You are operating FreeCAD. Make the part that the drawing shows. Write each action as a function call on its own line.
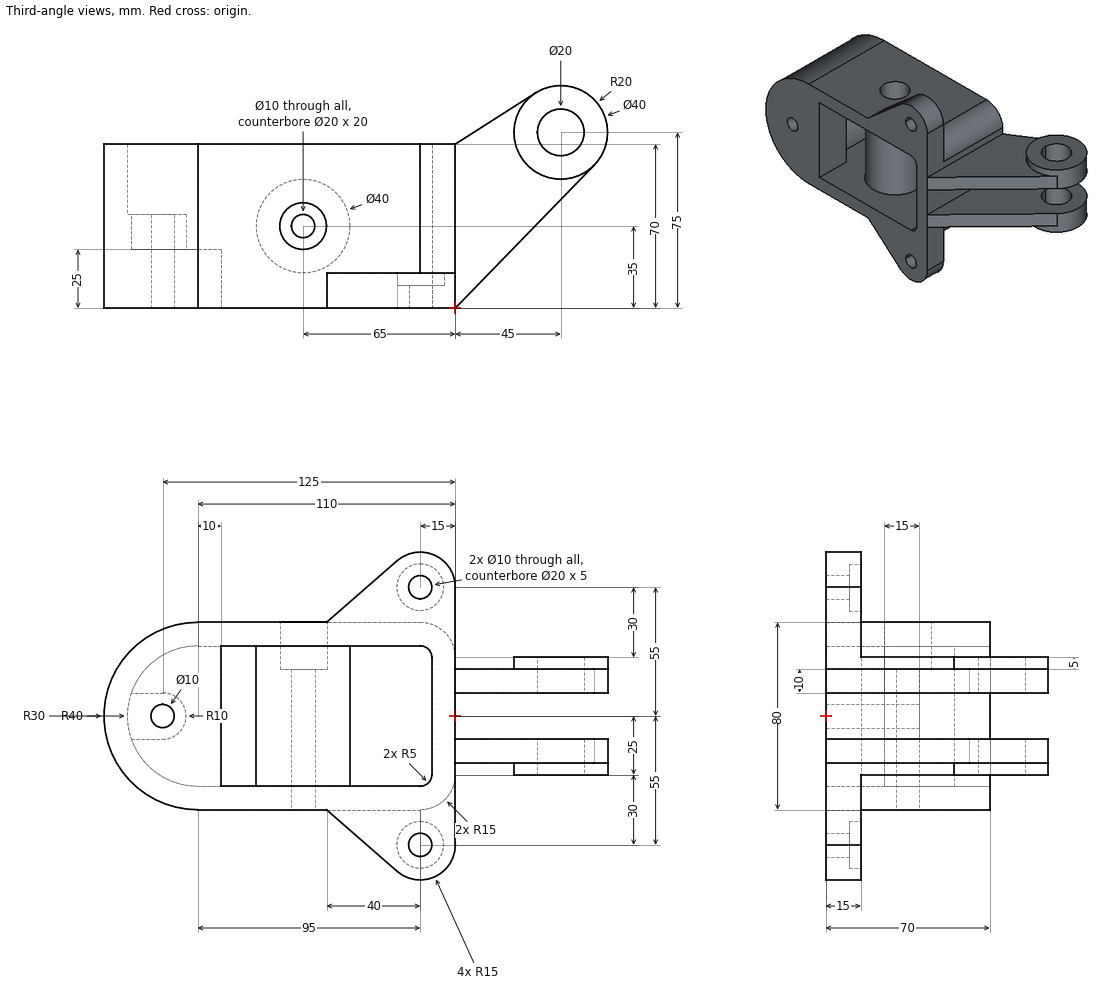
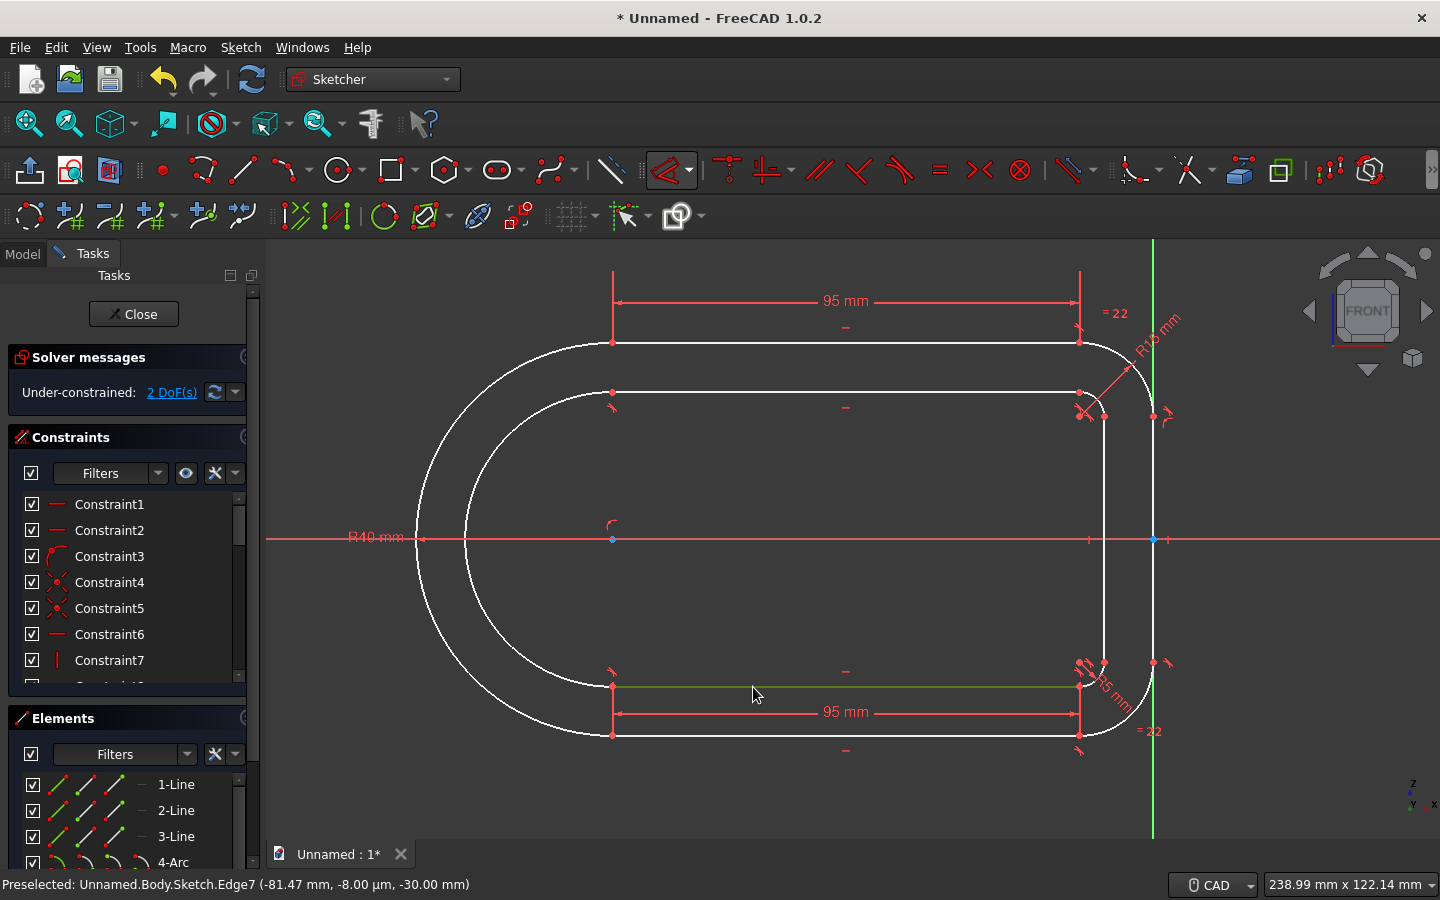
key(l)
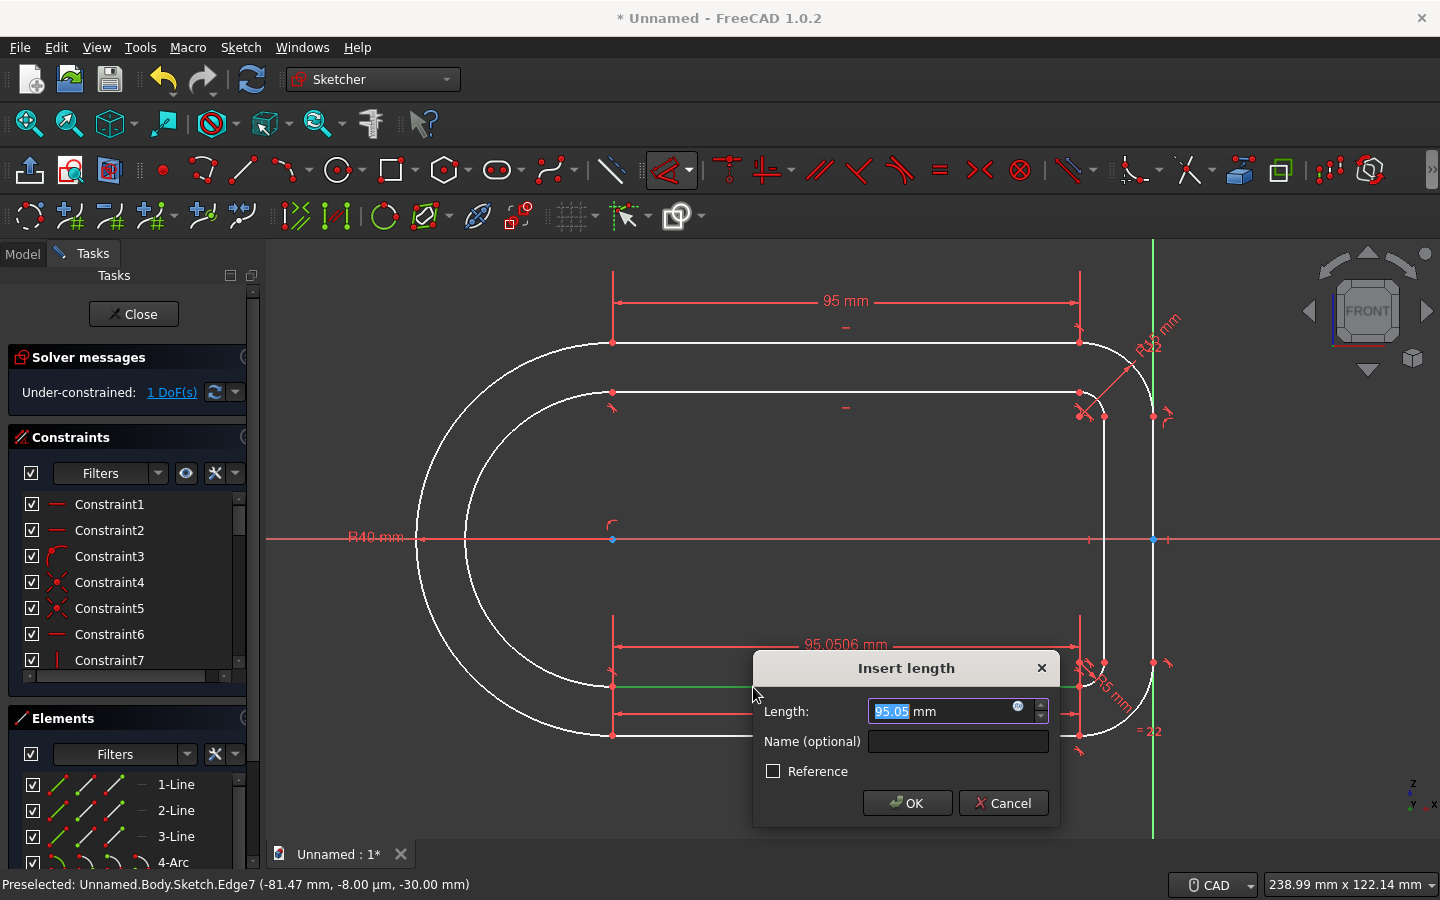
text(95)
key(Return)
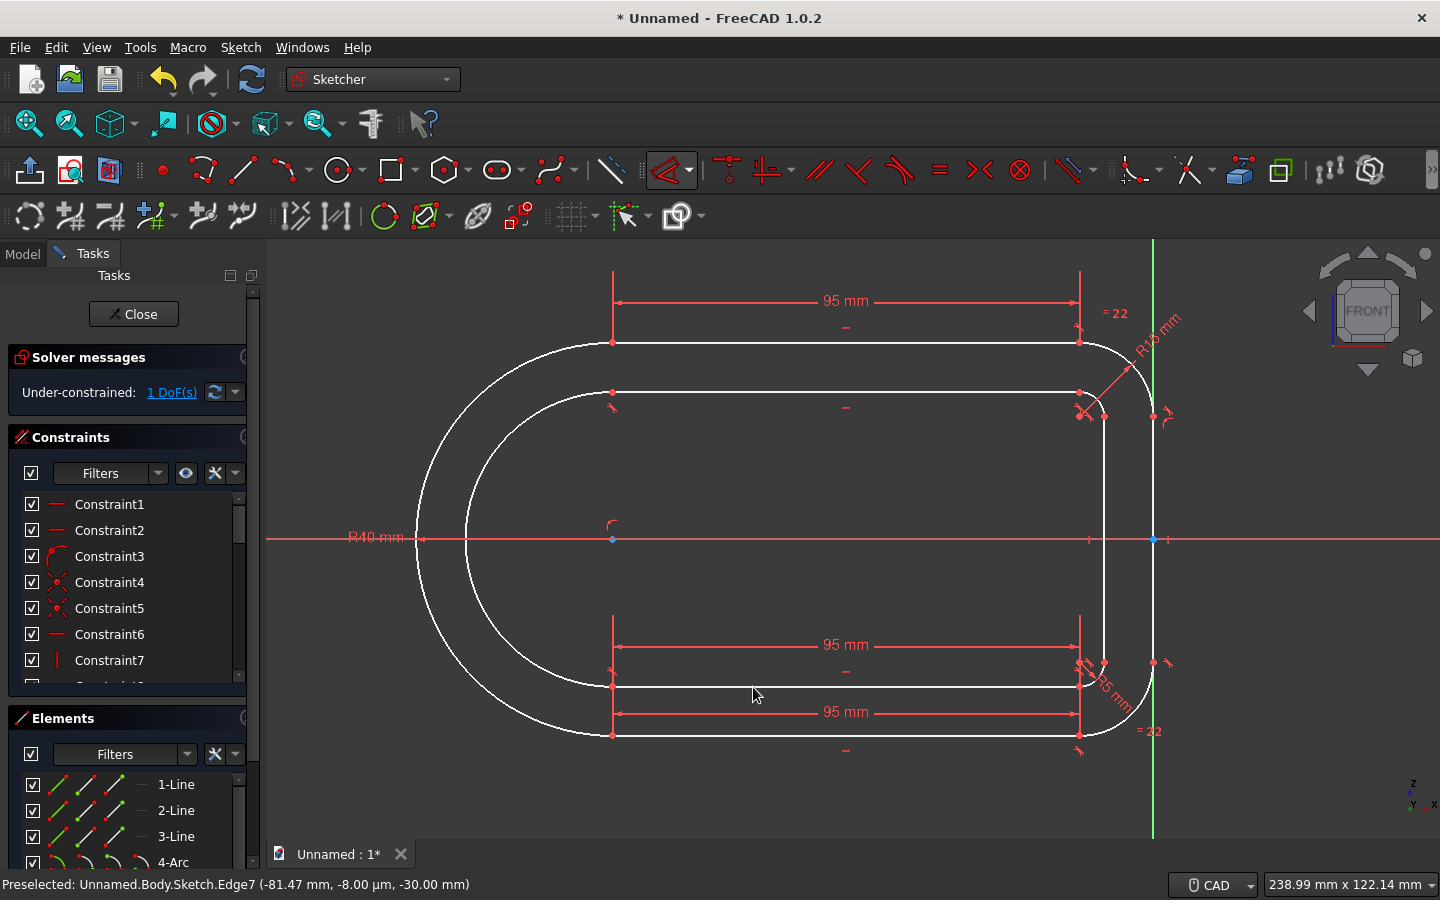
click(613, 539)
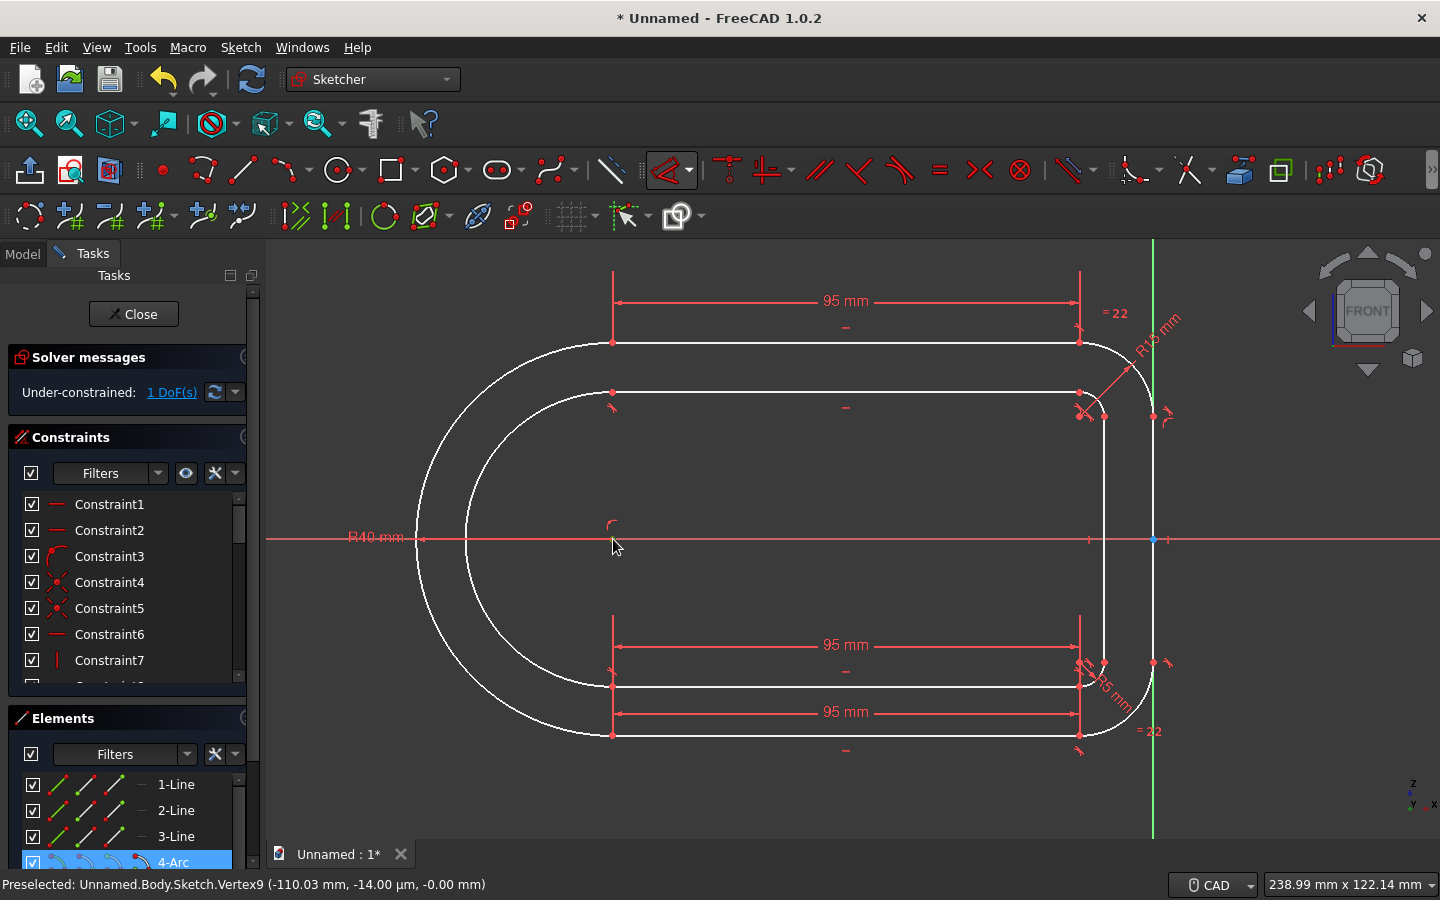
key(l)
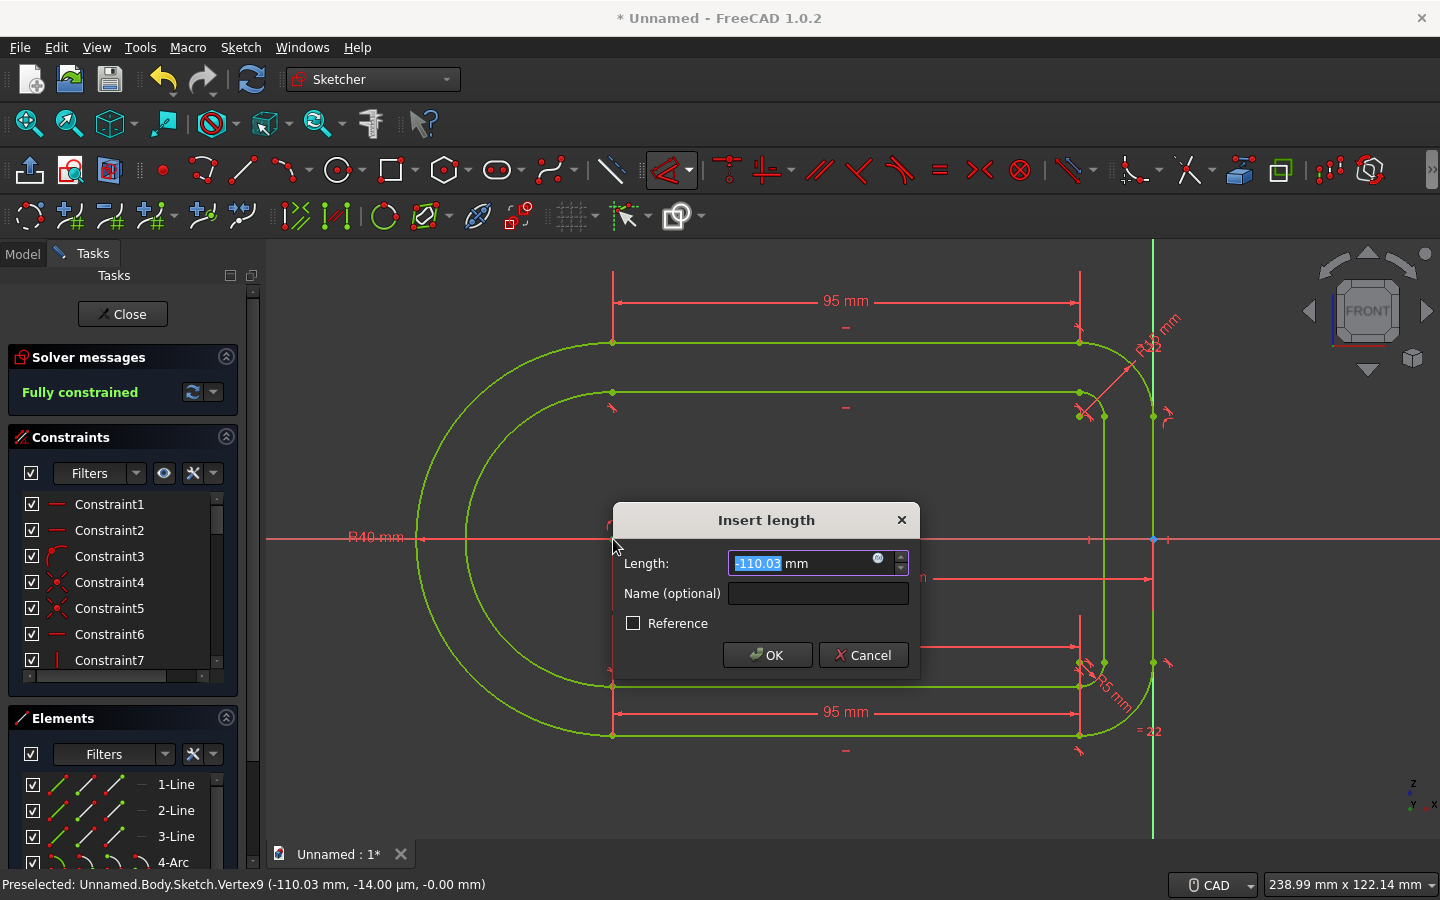
text(-110)
key(Return)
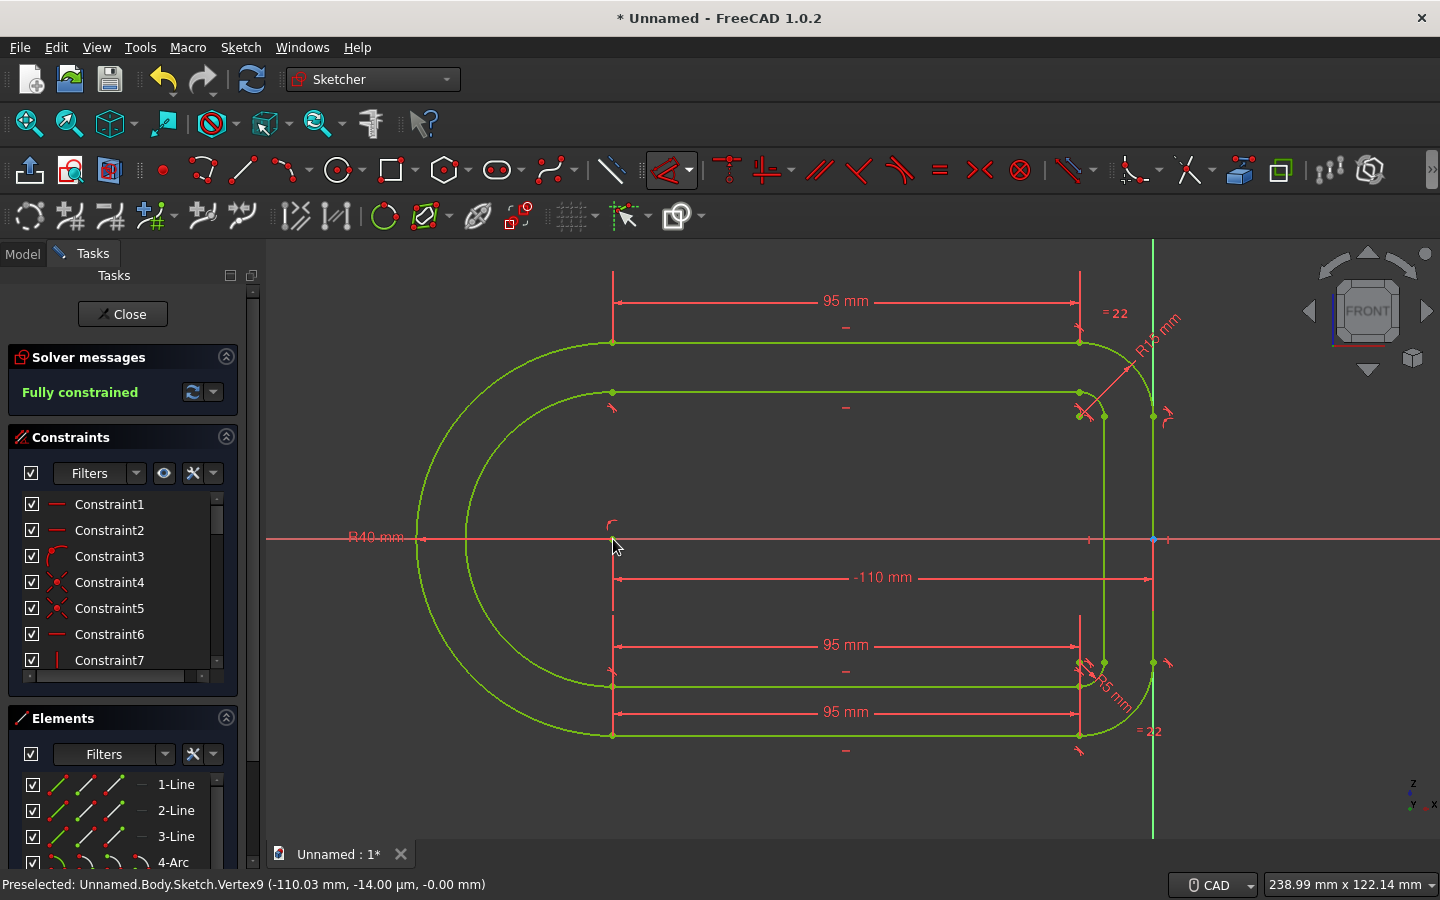
click(123, 314)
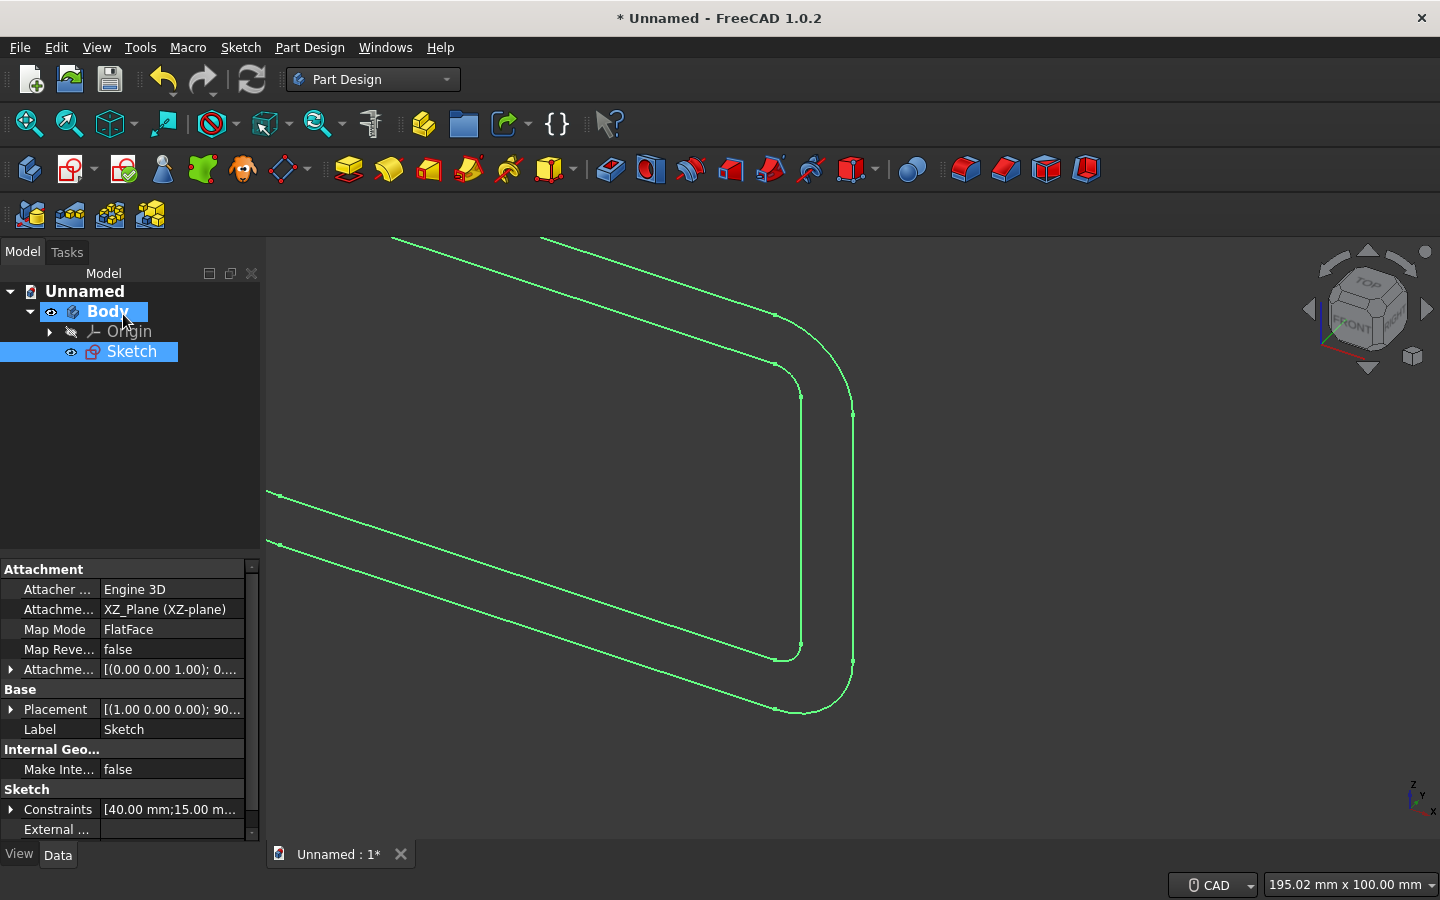
click(350, 170)